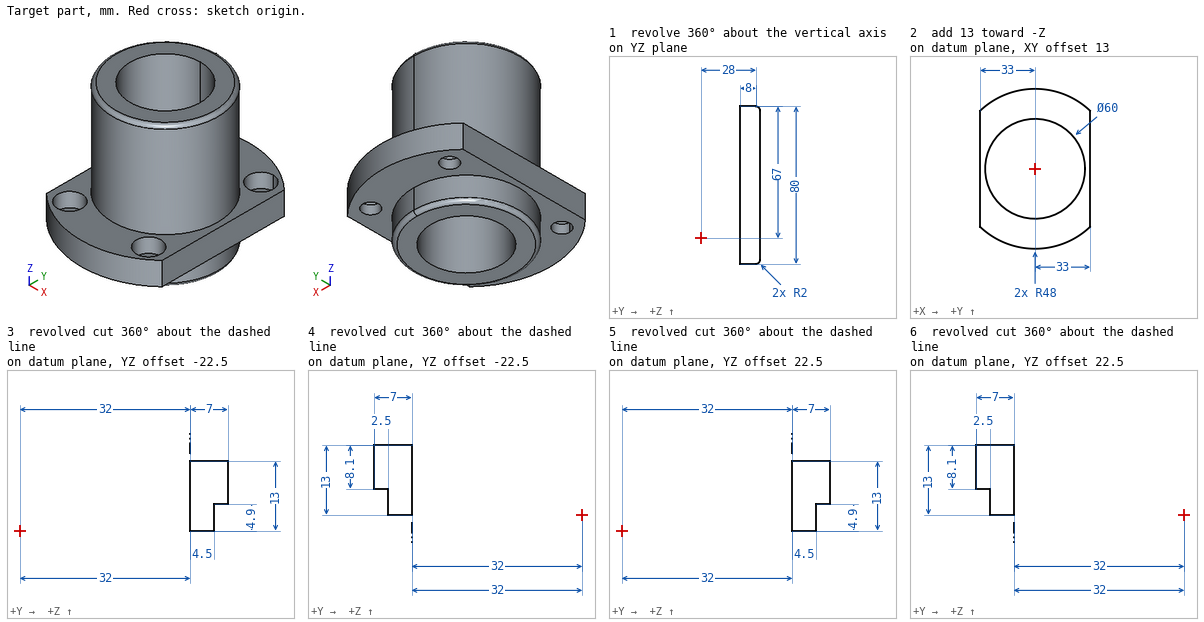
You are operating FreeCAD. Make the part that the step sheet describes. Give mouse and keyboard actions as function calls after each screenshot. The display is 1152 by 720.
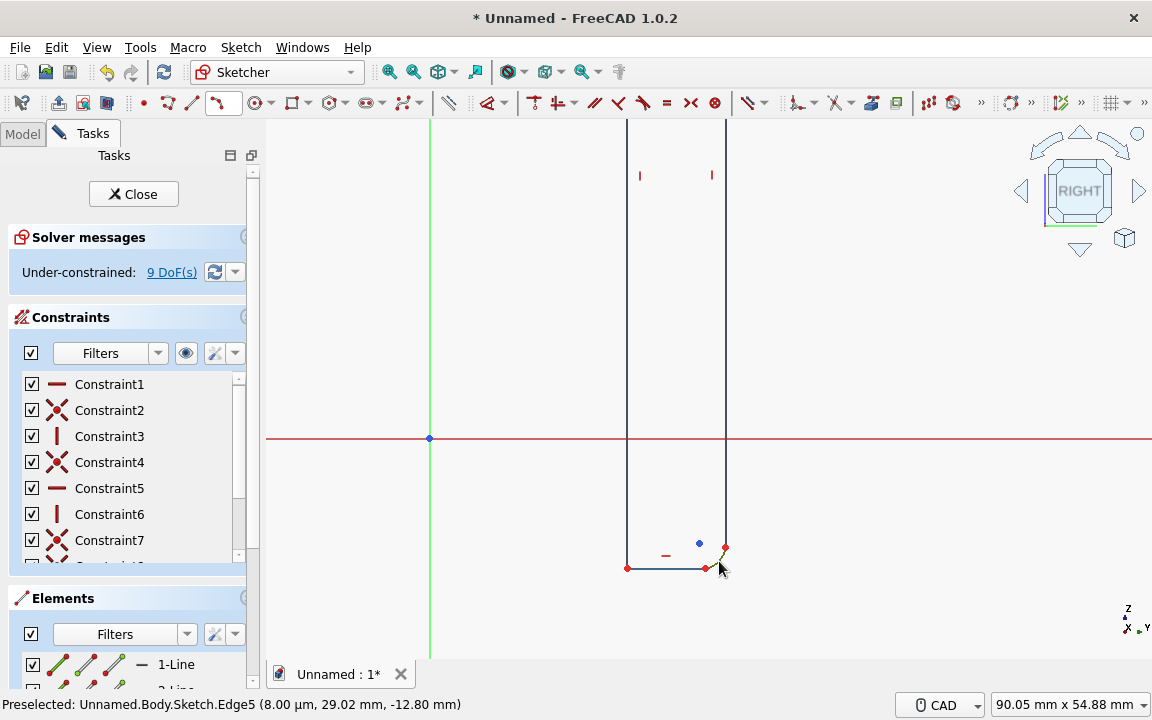
click(644, 104)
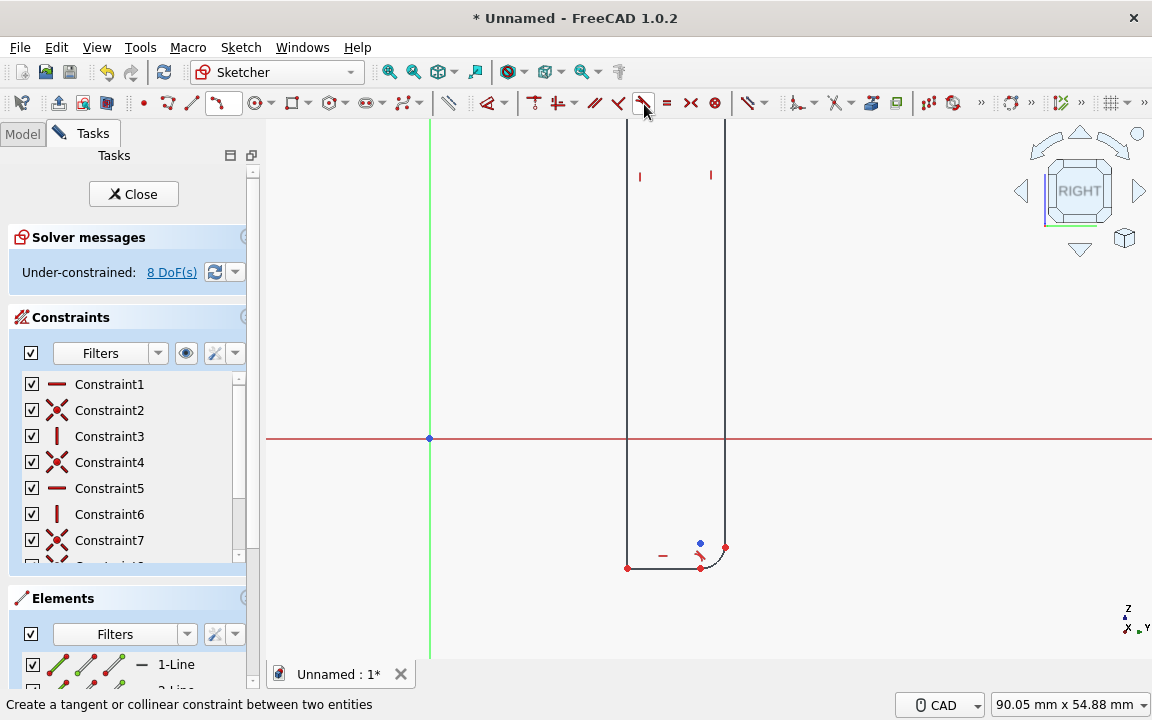
click(725, 324)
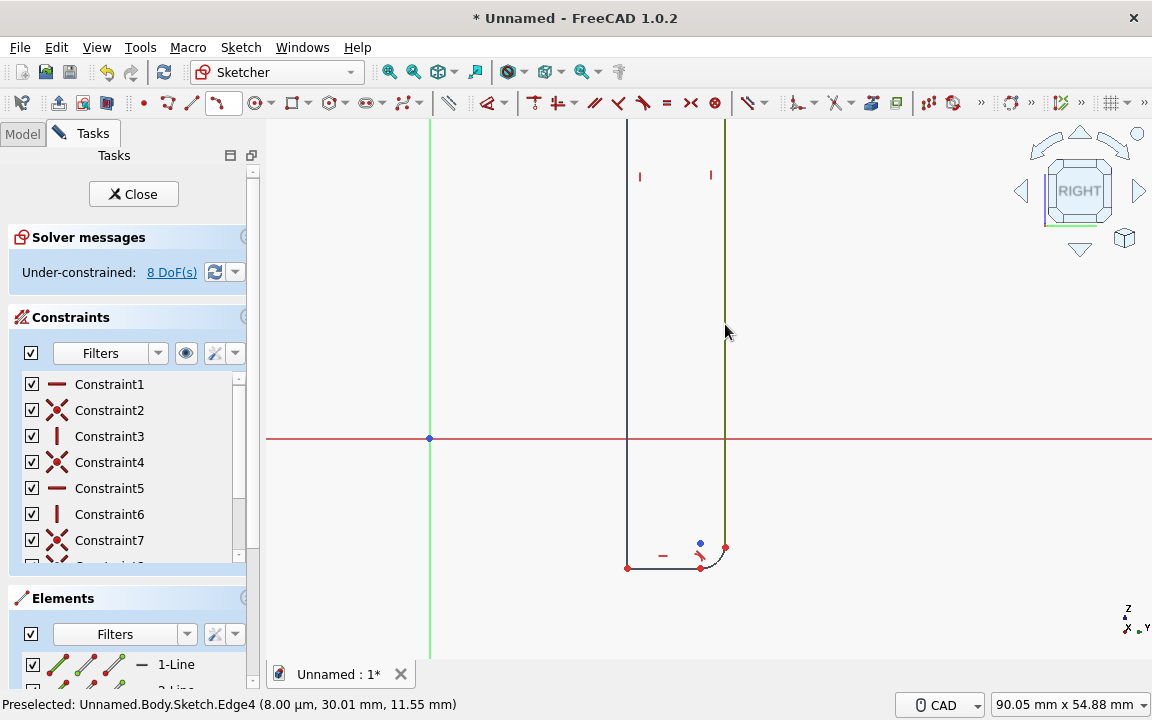
scroll(710, 567, up, 2)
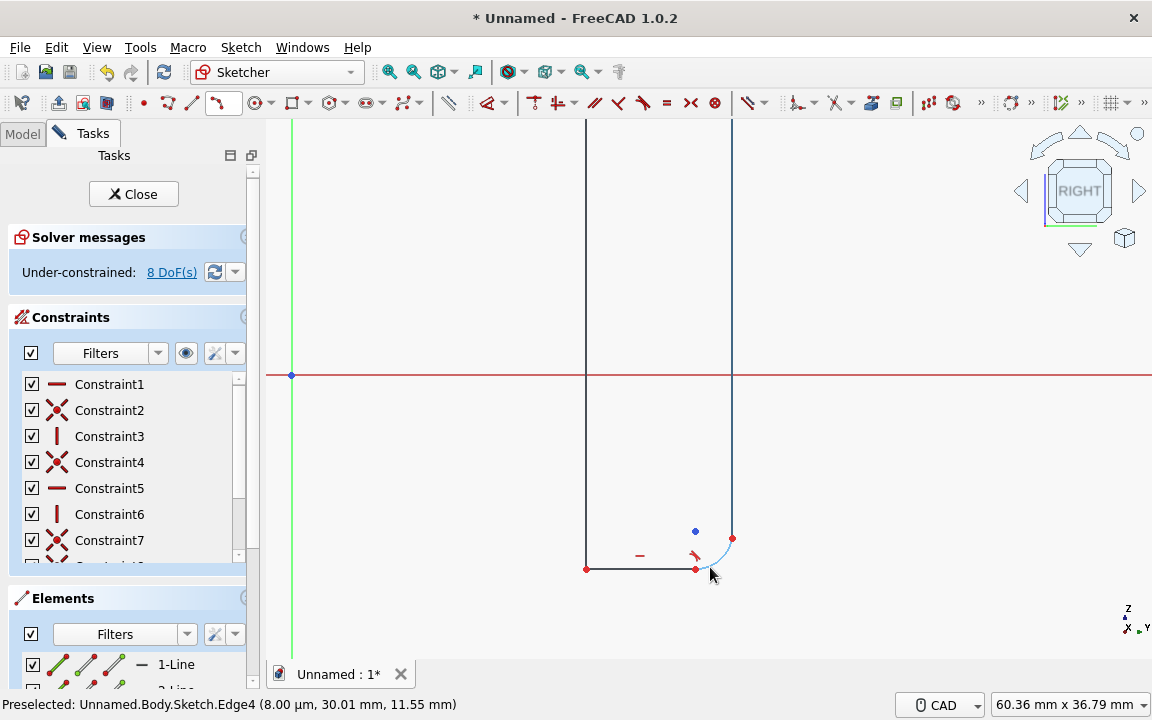
click(710, 566)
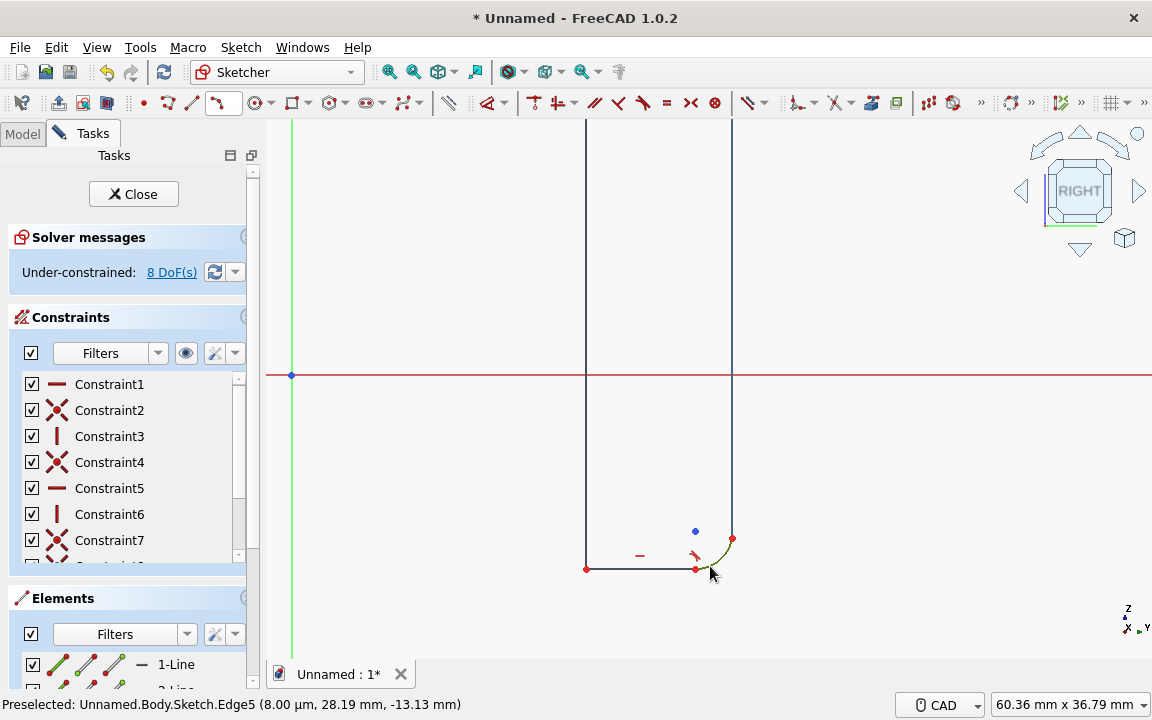
click(644, 104)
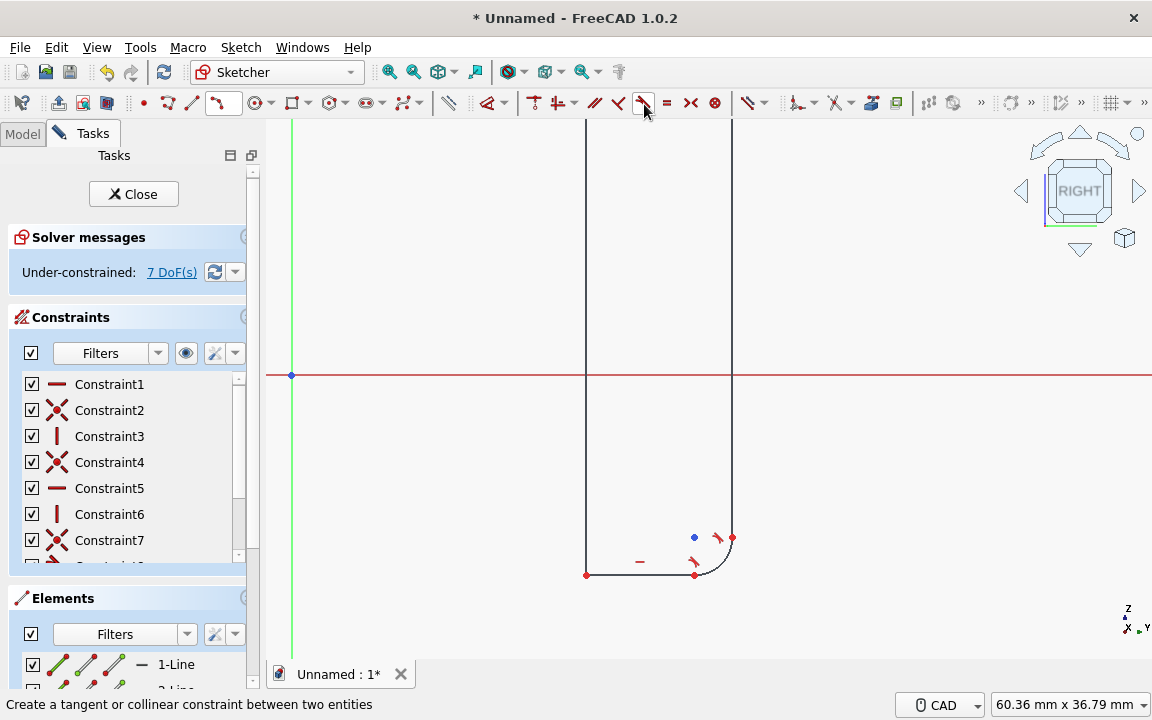
scroll(696, 566, down, 6)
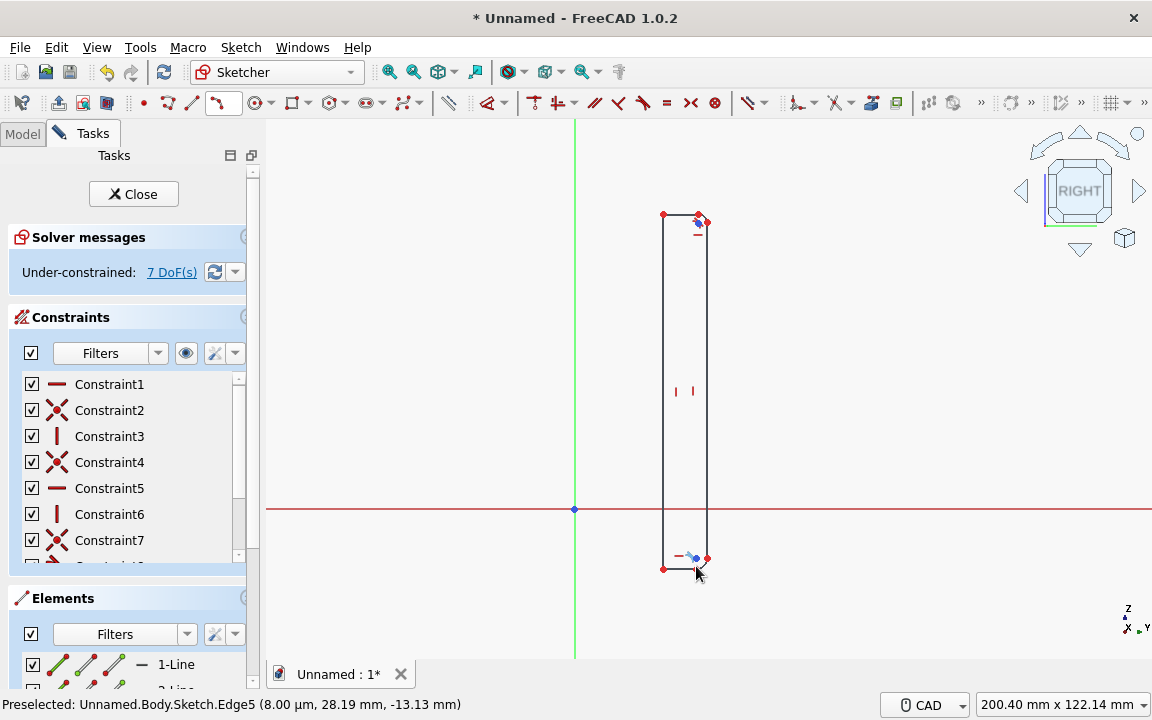
click(707, 457)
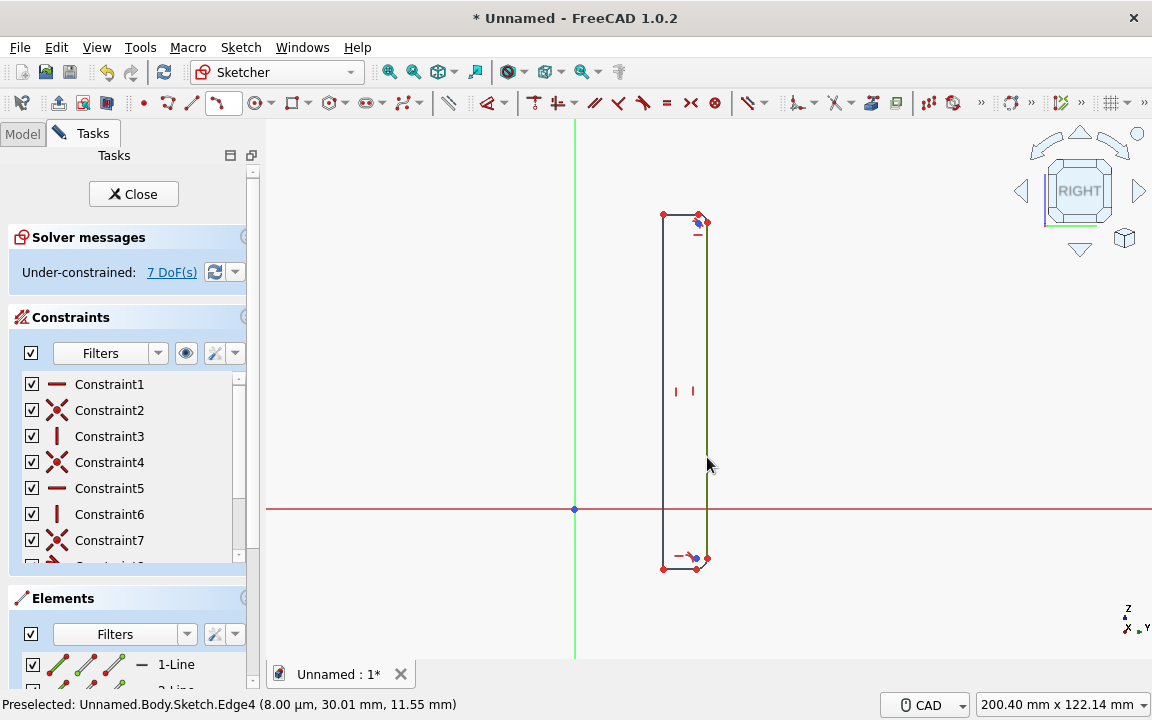
scroll(705, 217, up, 5)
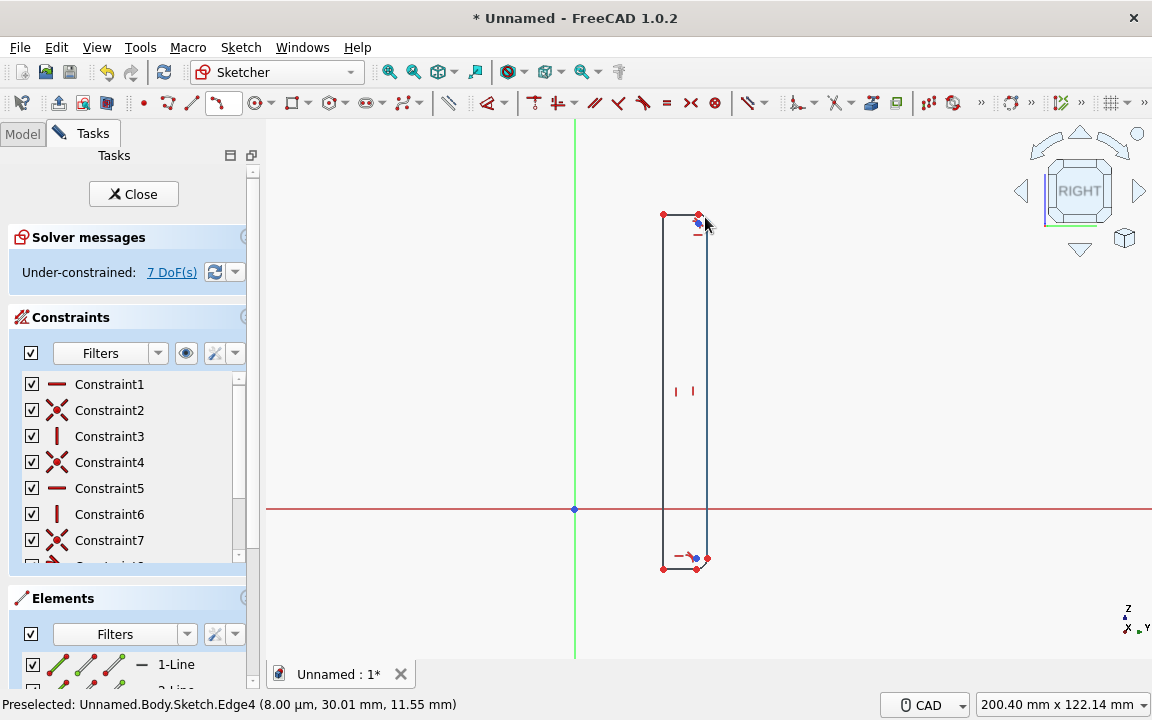
click(703, 216)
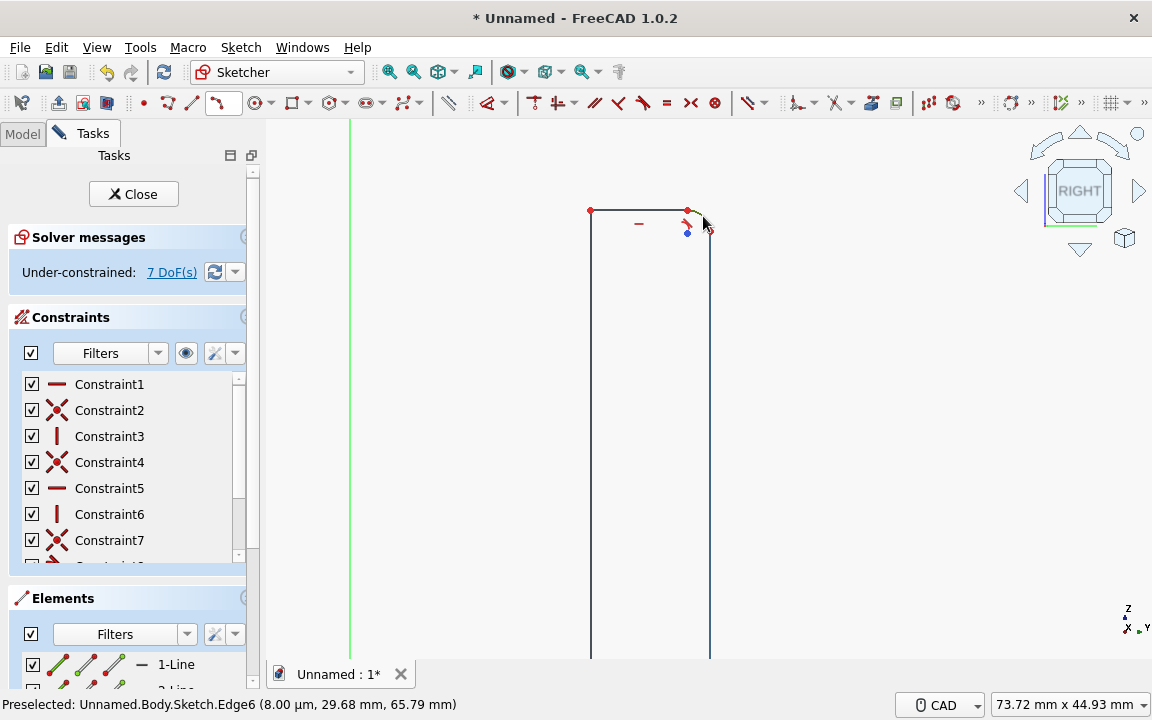
click(644, 104)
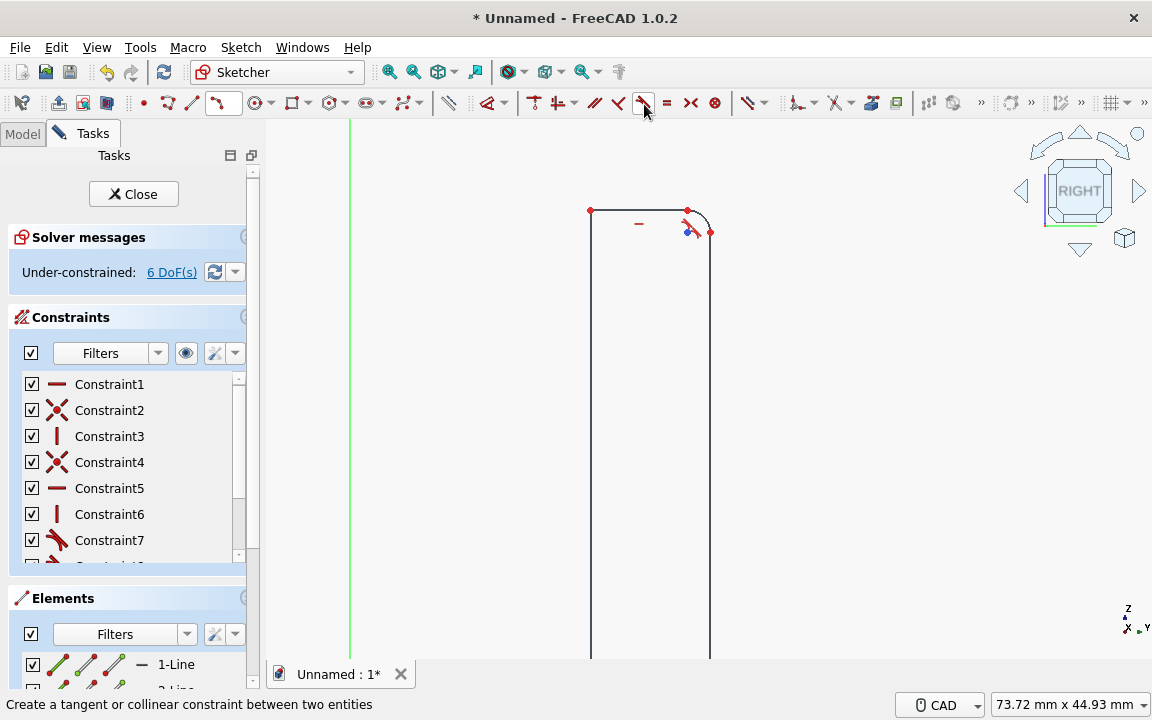
scroll(705, 216, down, 5)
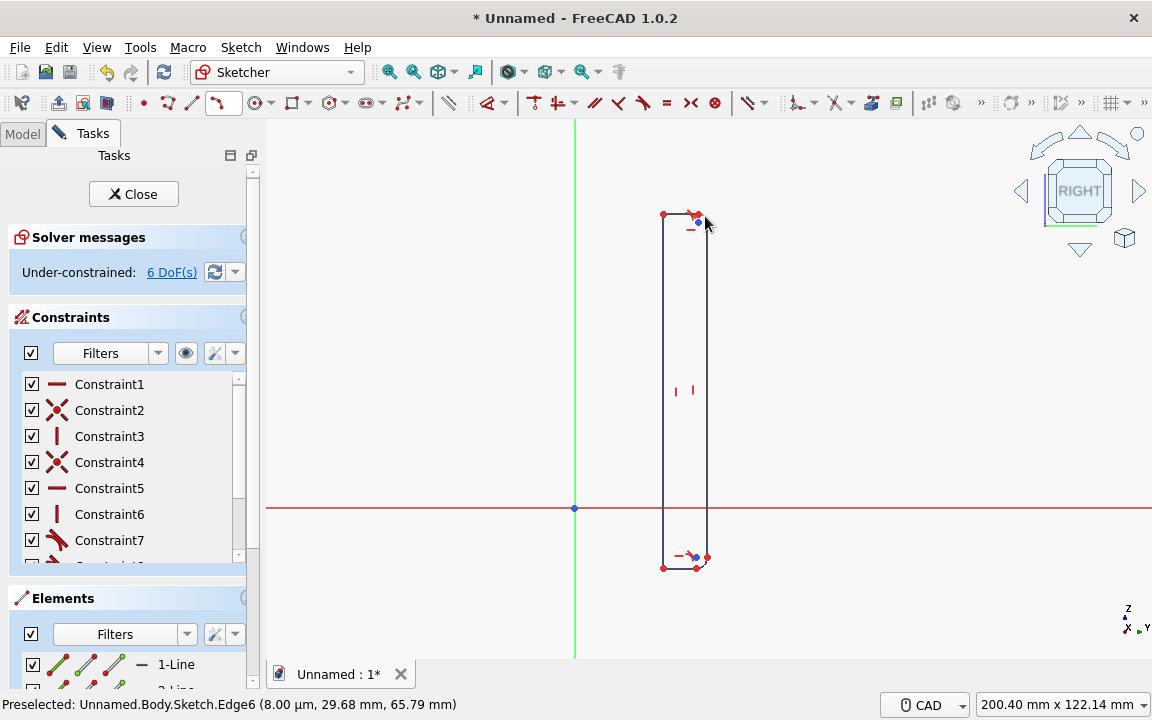
scroll(701, 567, up, 5)